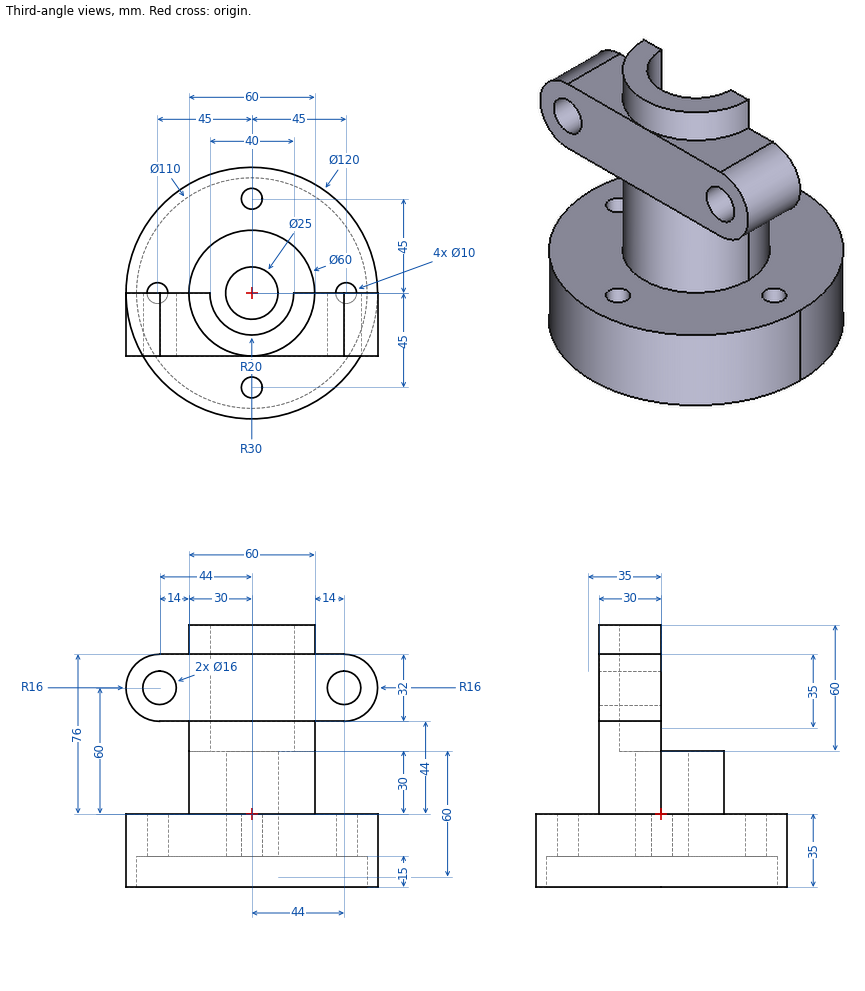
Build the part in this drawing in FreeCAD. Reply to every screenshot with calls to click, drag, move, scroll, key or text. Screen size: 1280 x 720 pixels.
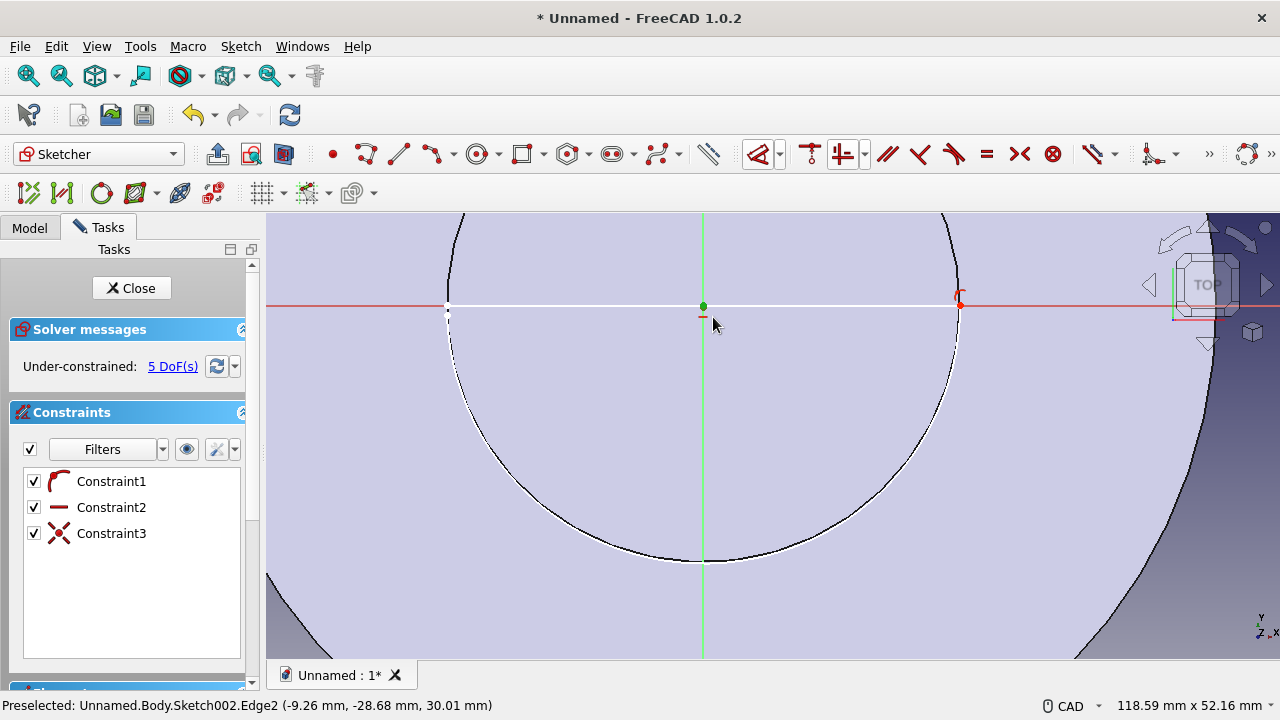
click(810, 154)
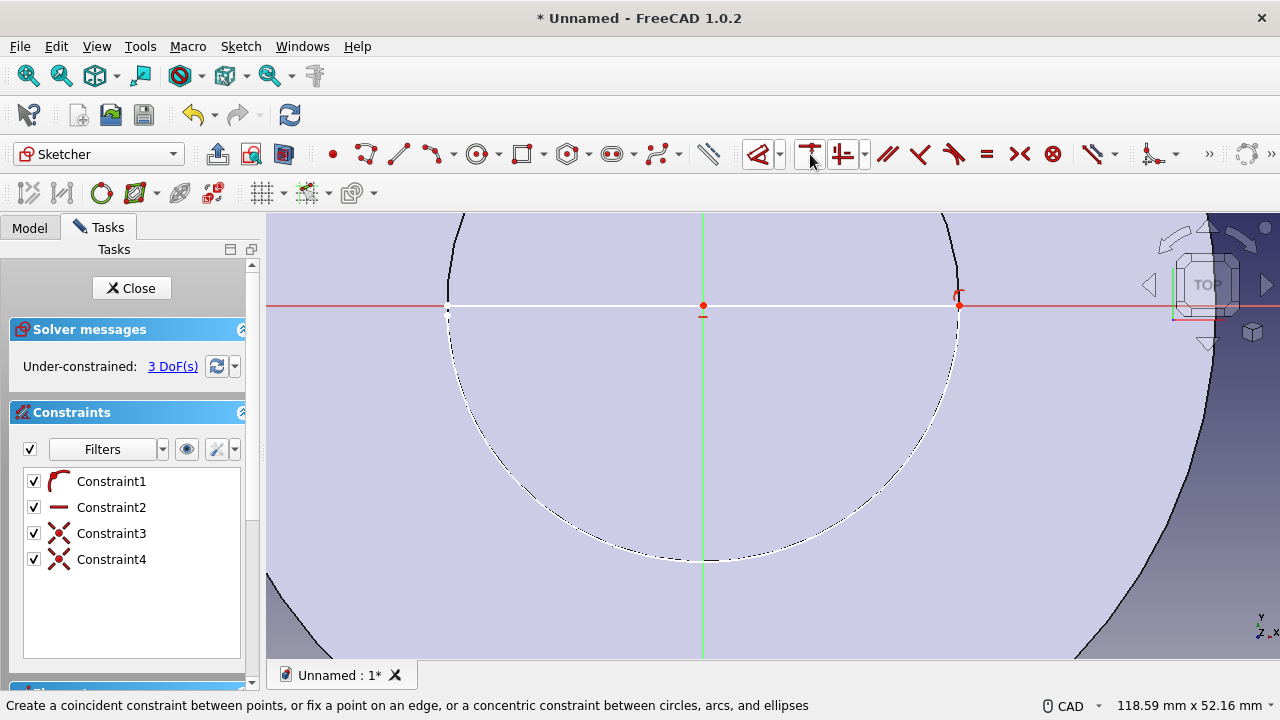
click(758, 154)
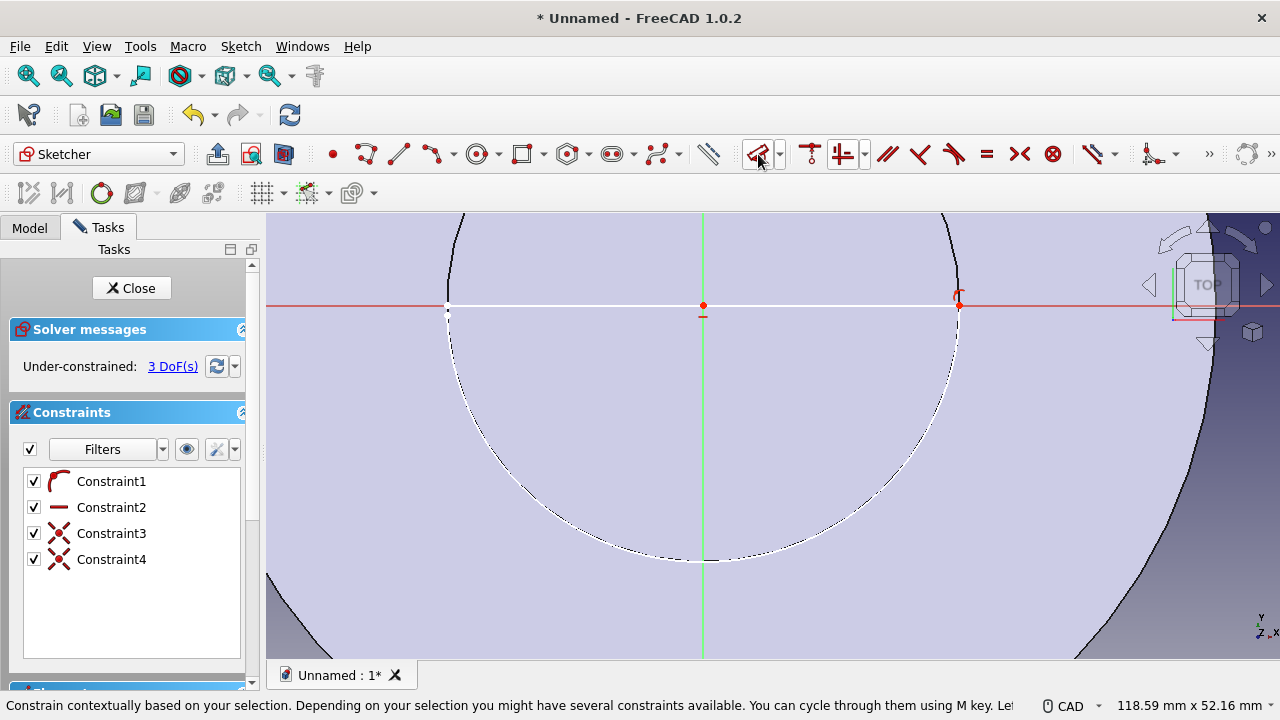
click(558, 517)
click(540, 543)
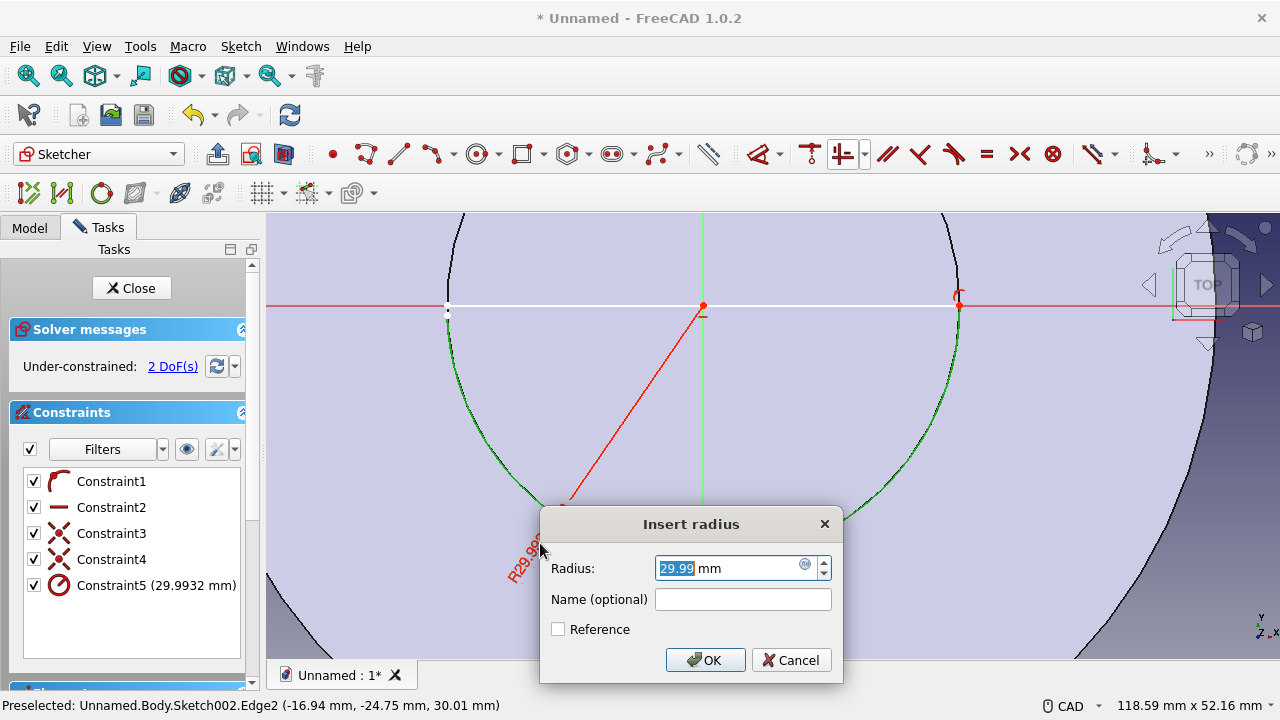
text(30)
key(Return)
key(Escape)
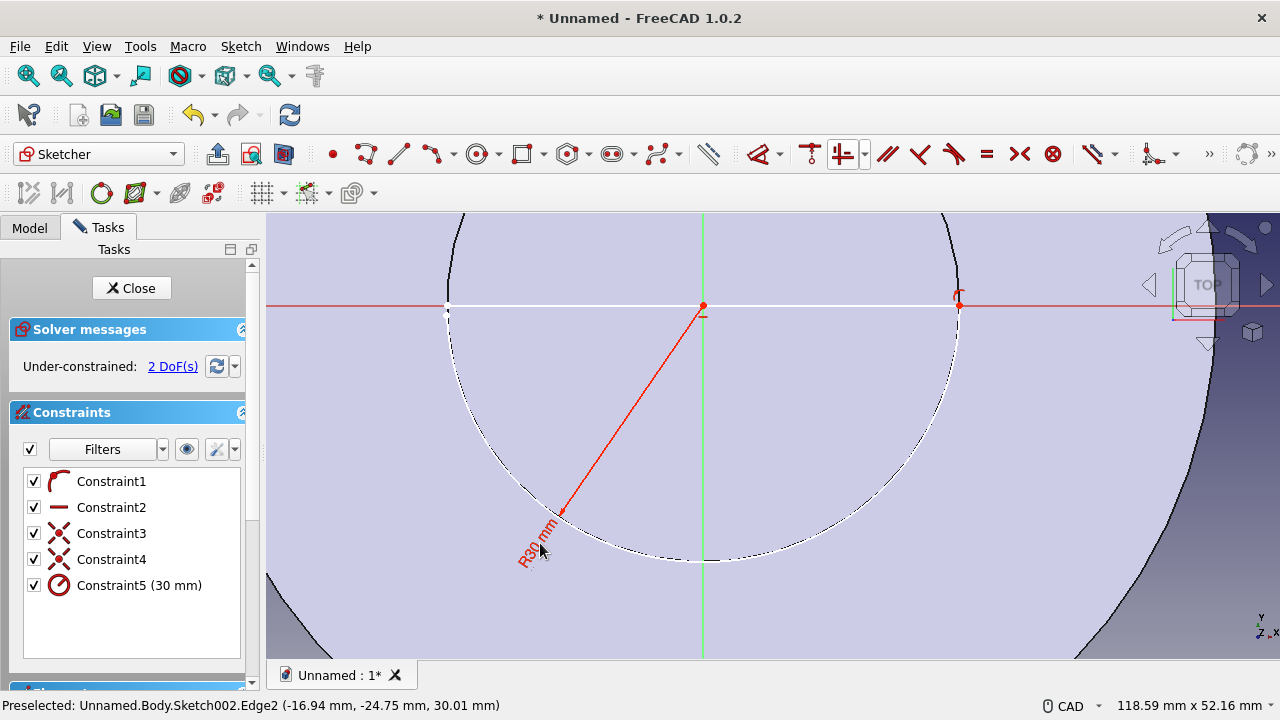
click(447, 316)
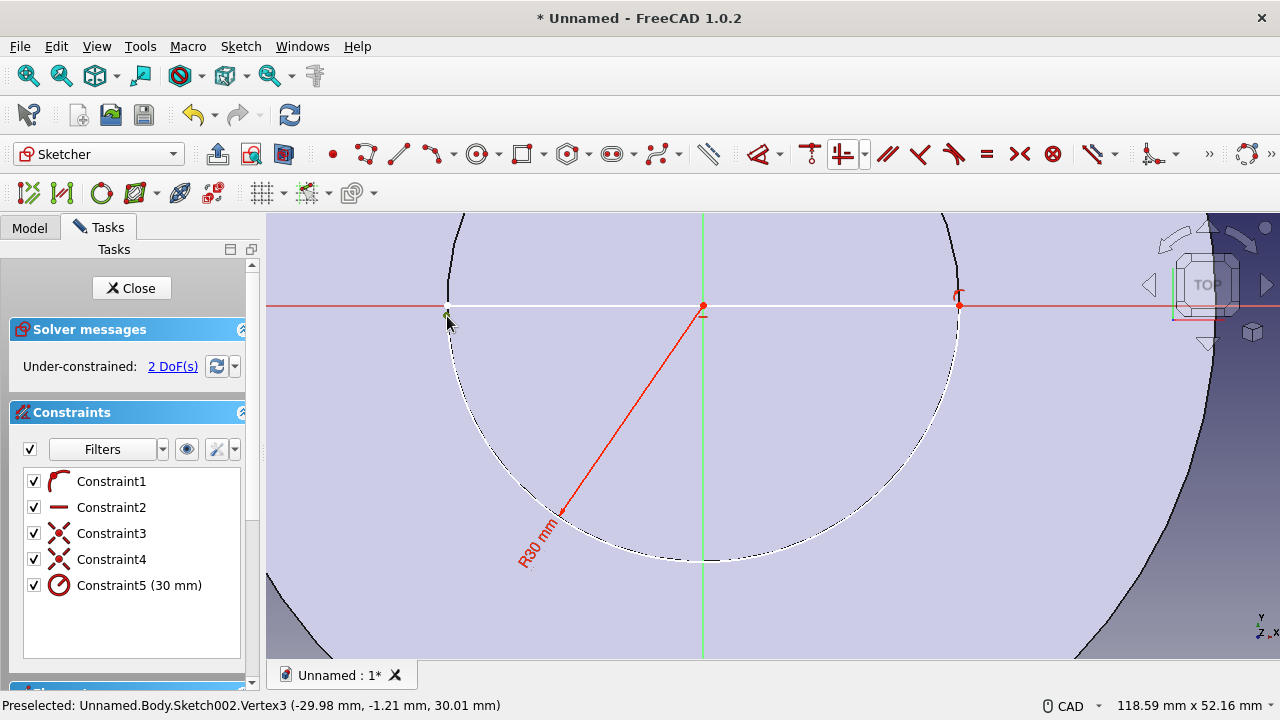
click(353, 306)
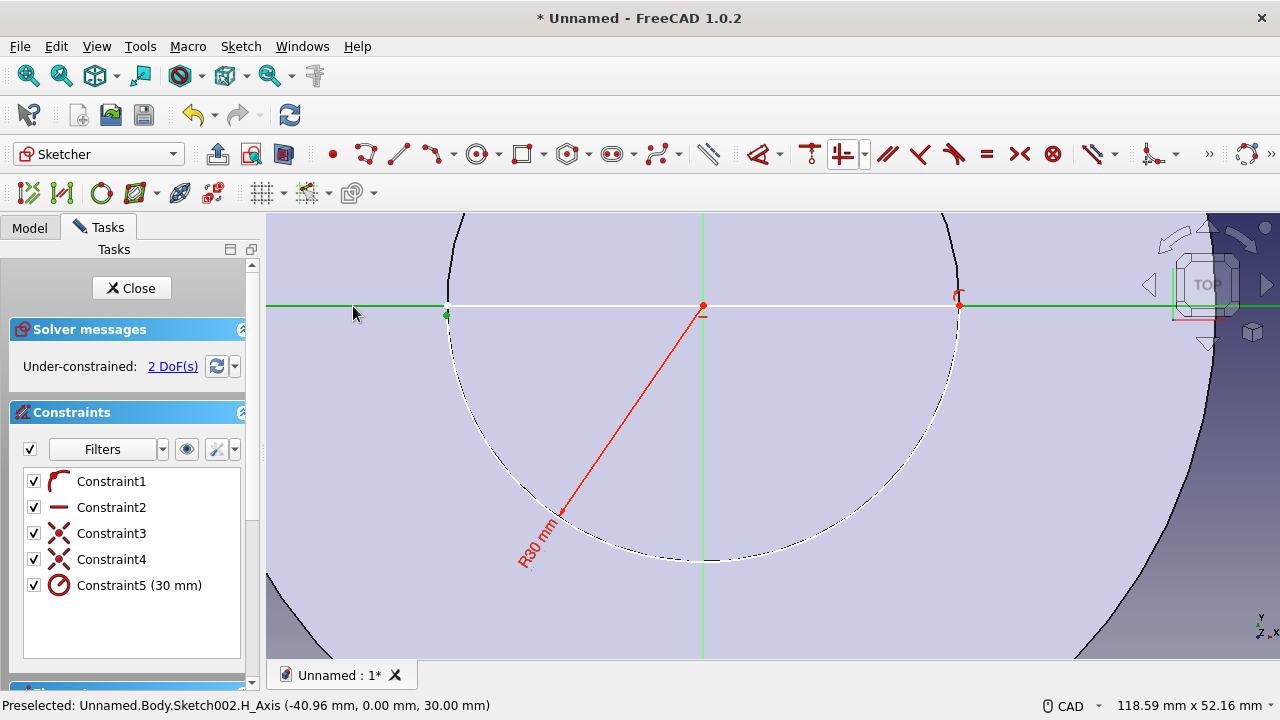
click(810, 154)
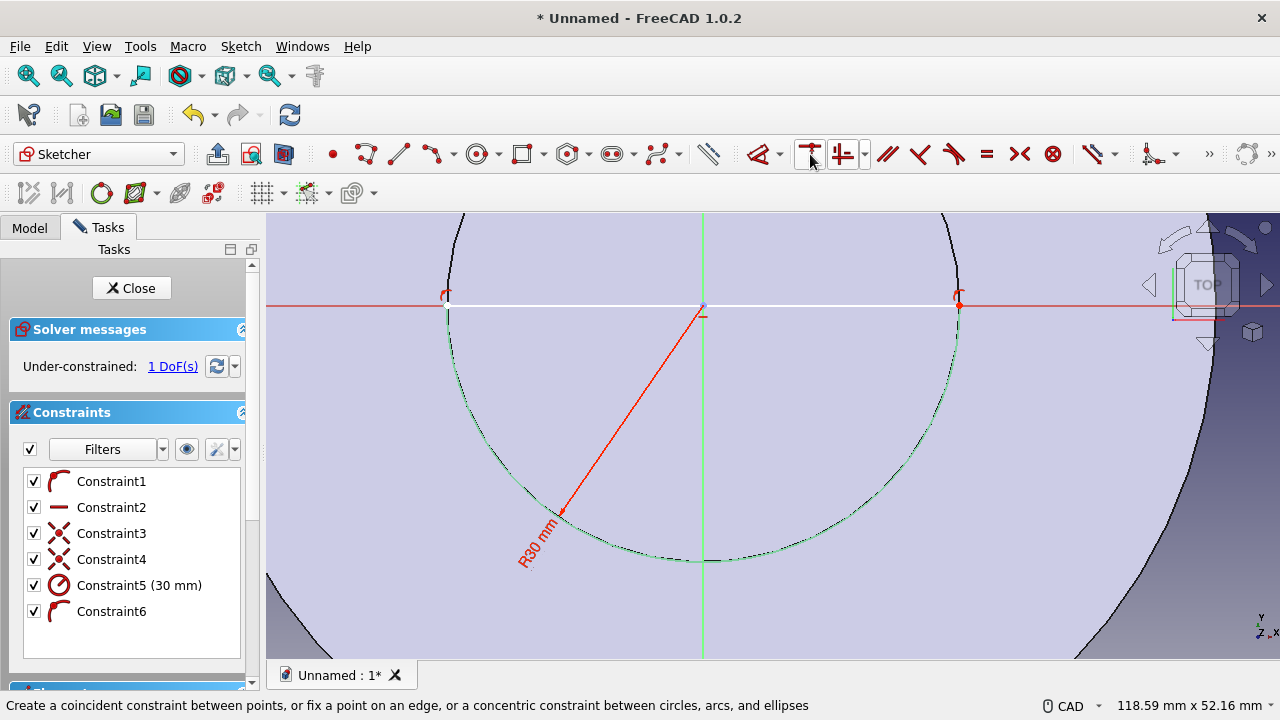
click(758, 154)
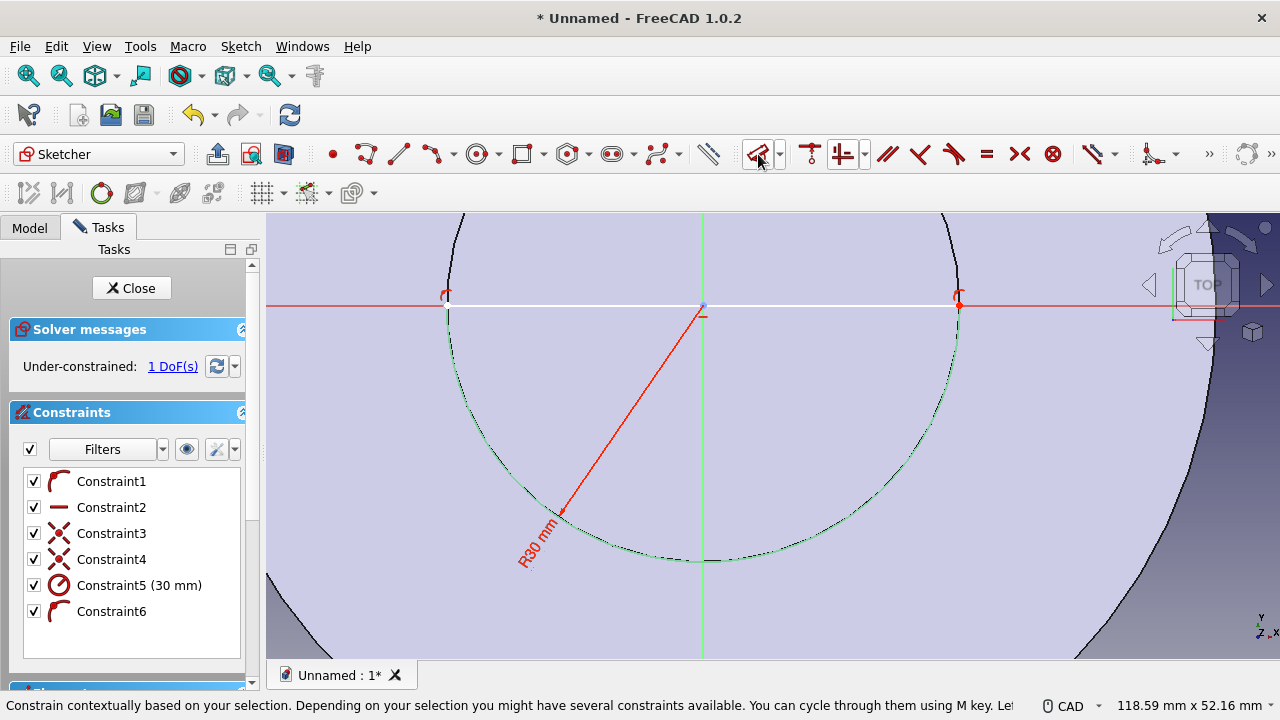
click(806, 306)
click(585, 272)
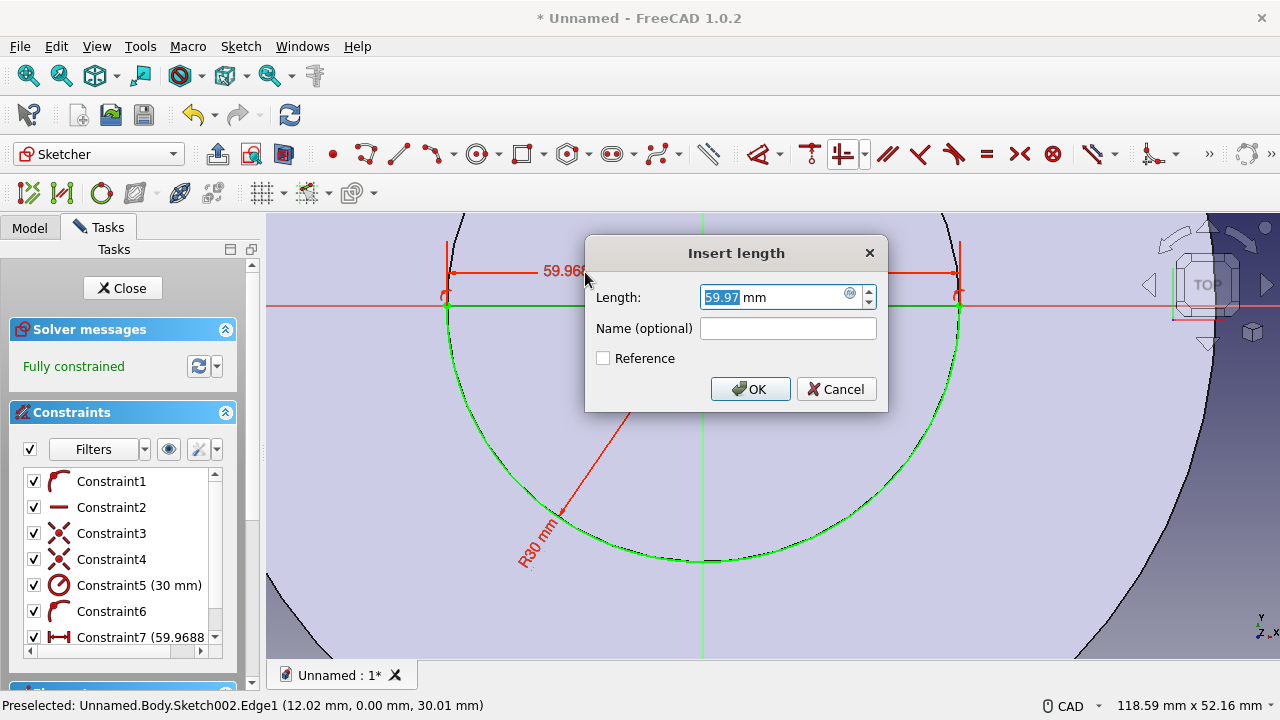
text(60)
key(Return)
key(Escape)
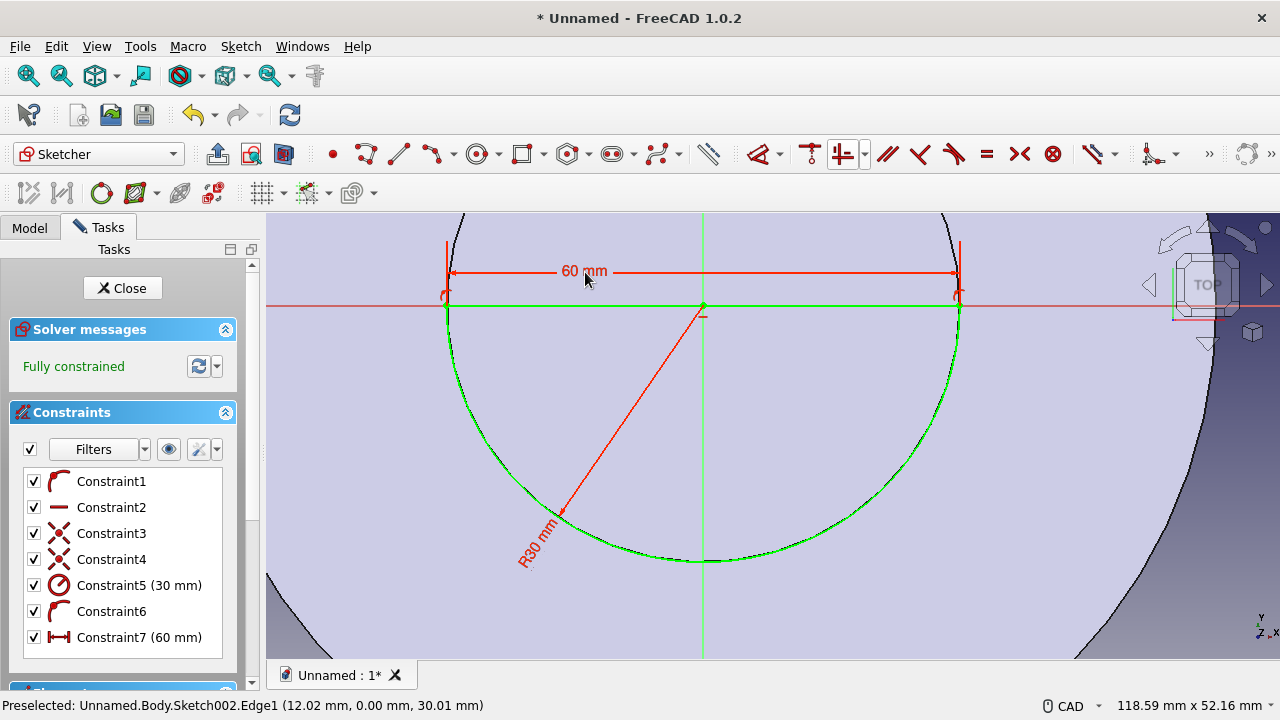
click(123, 288)